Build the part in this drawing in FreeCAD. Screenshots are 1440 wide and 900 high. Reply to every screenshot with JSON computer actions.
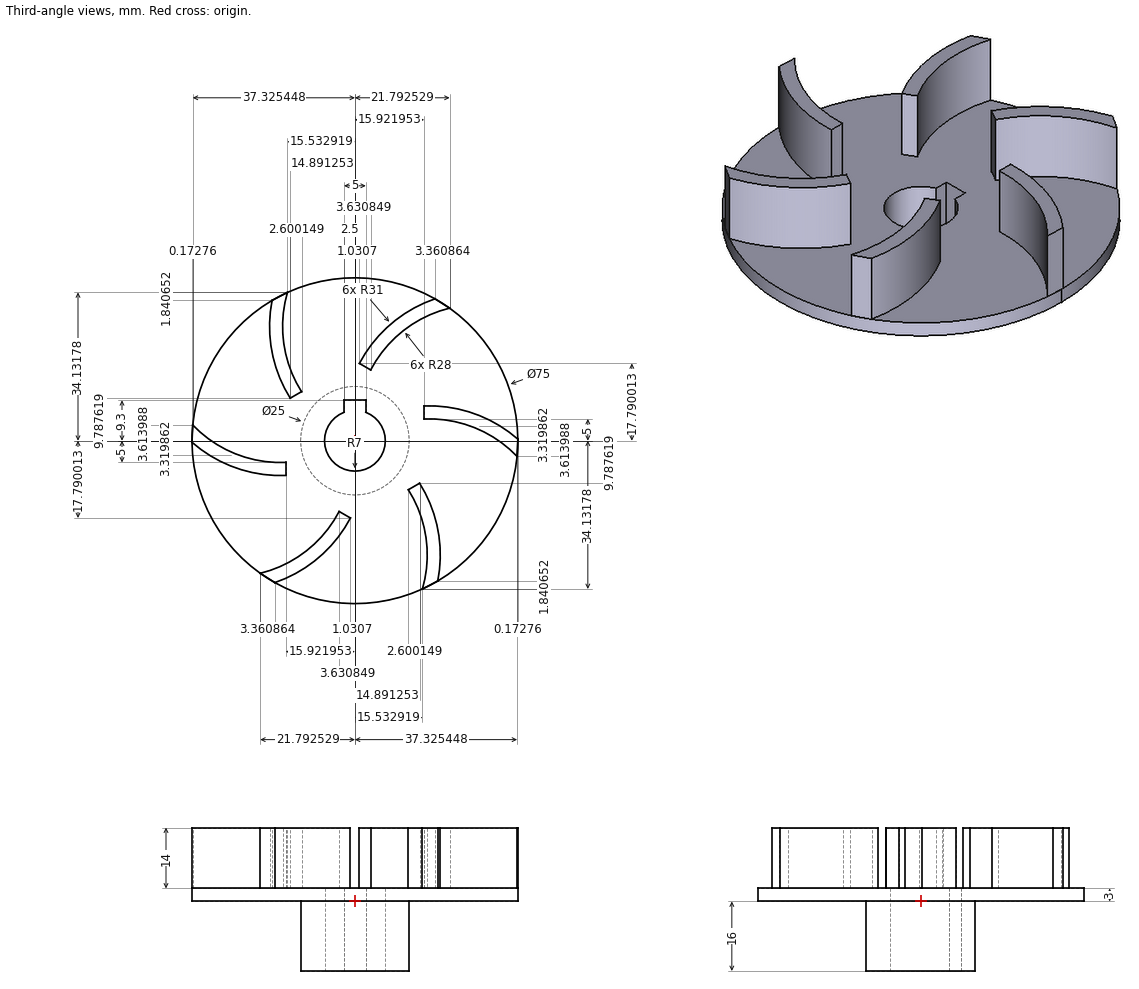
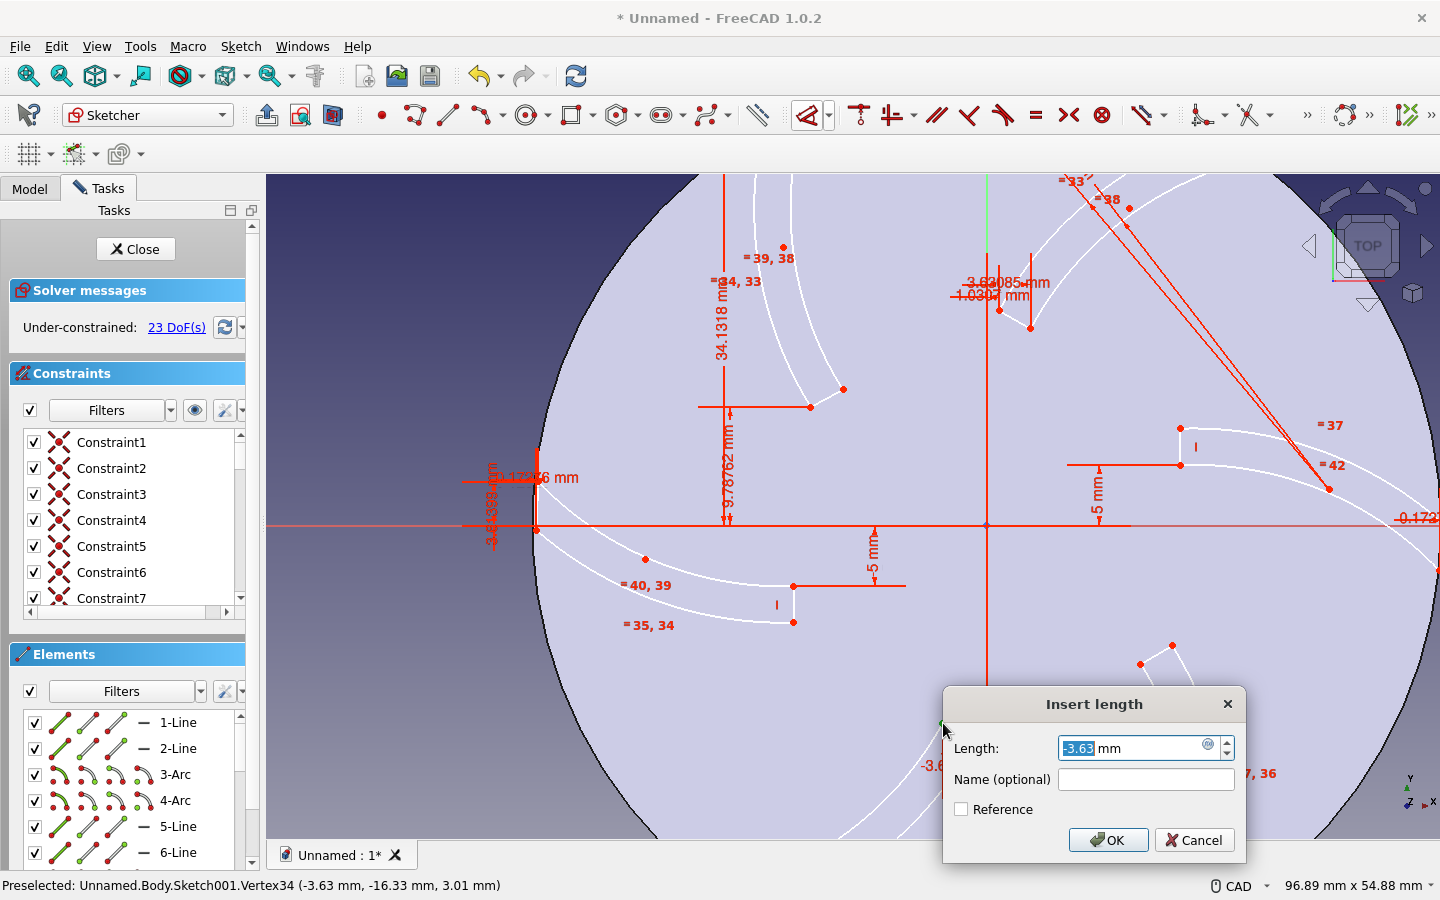
{"action": "type", "text": "-3.630849"}
{"action": "key", "text": "Return"}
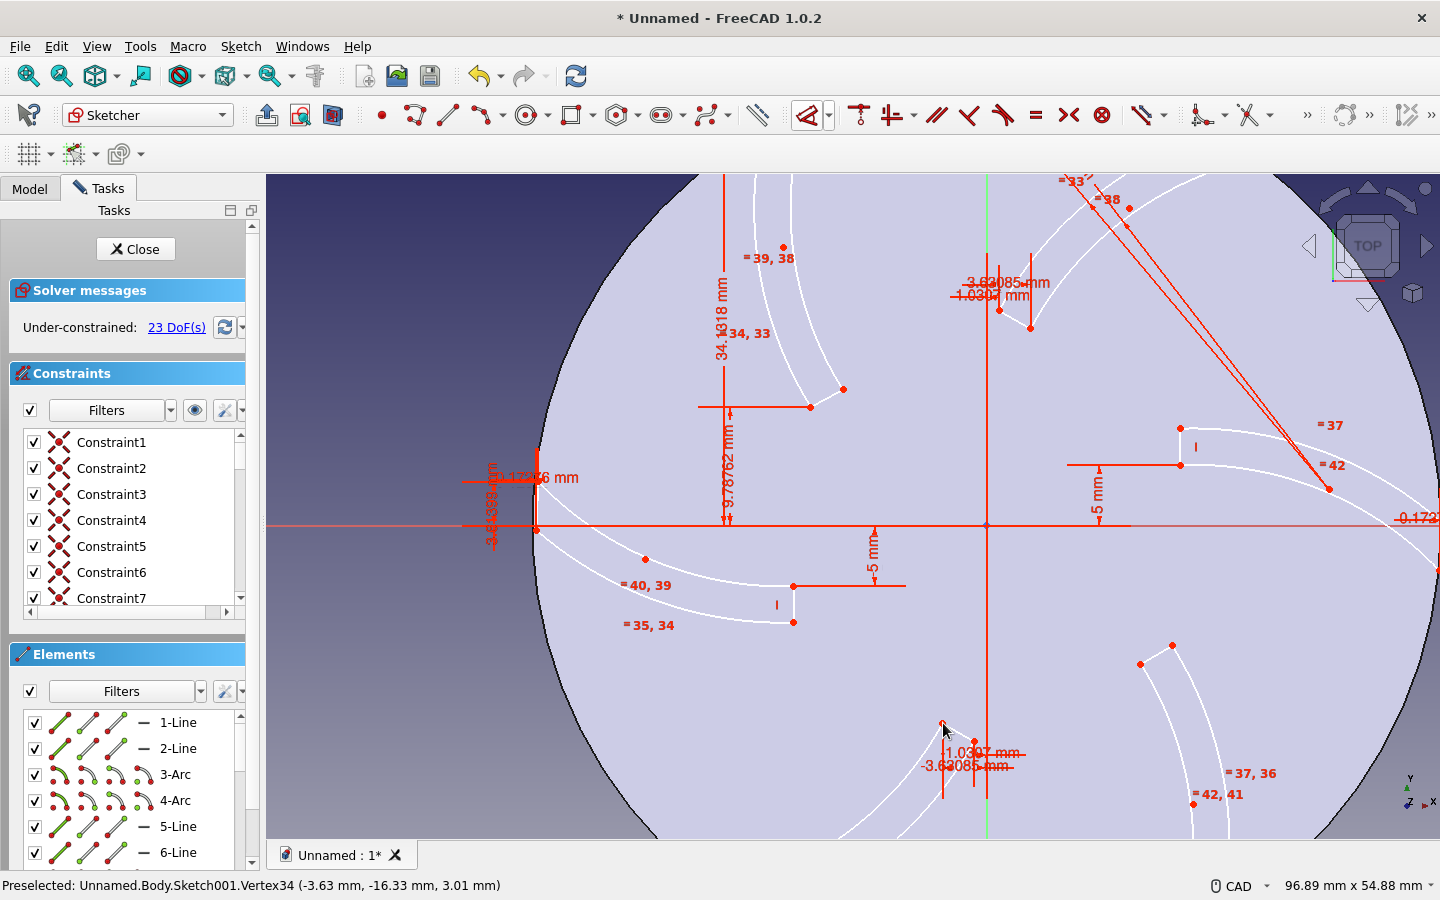
{"action": "scroll", "coordinate": [539, 483], "scroll_direction": "down", "scroll_amount": 3}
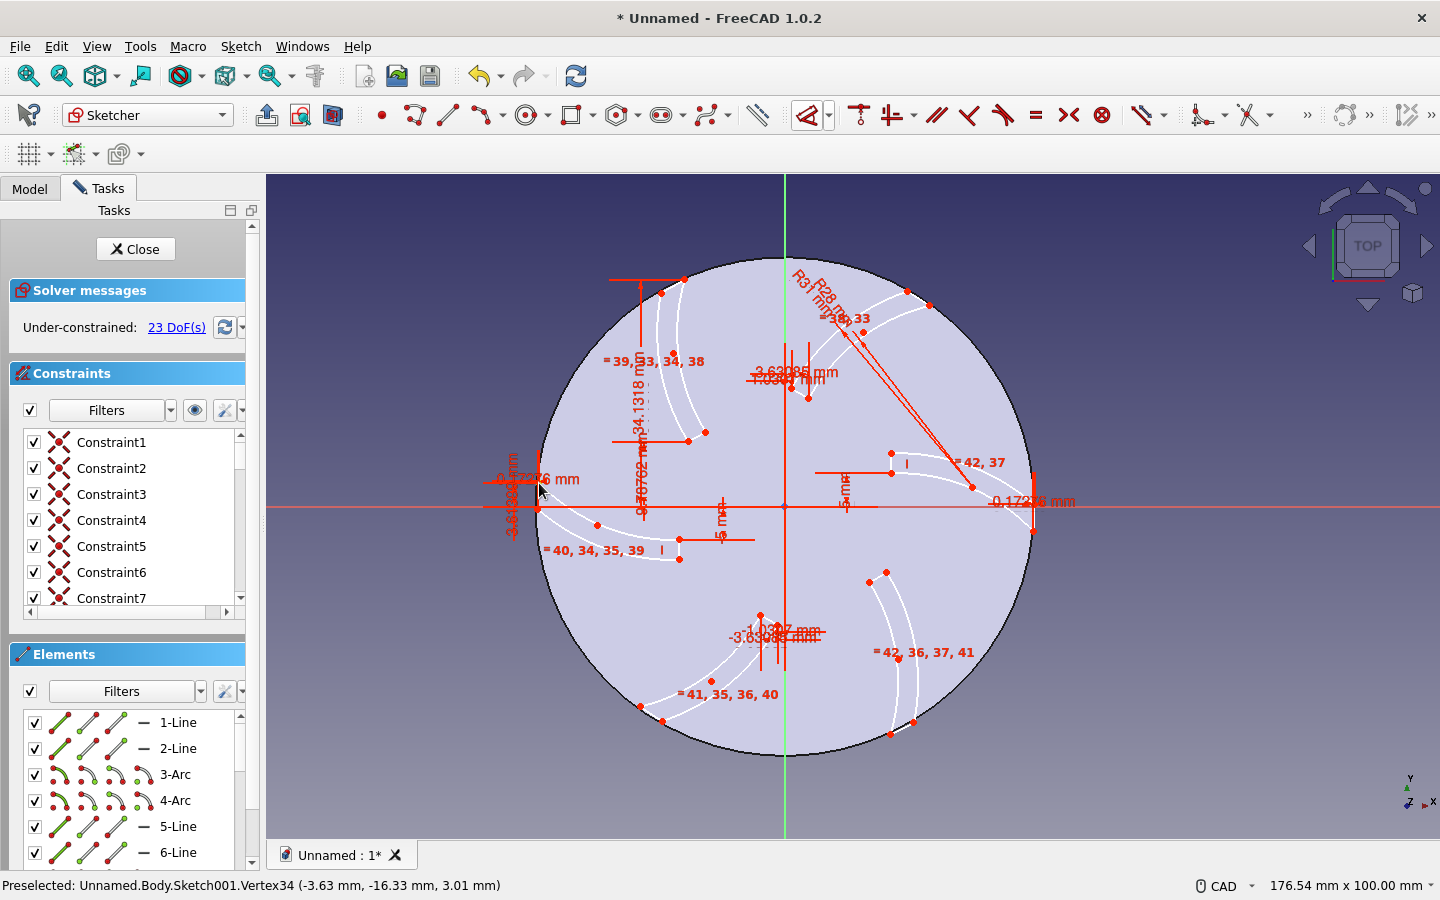
{"action": "left_click", "coordinate": [890, 735]}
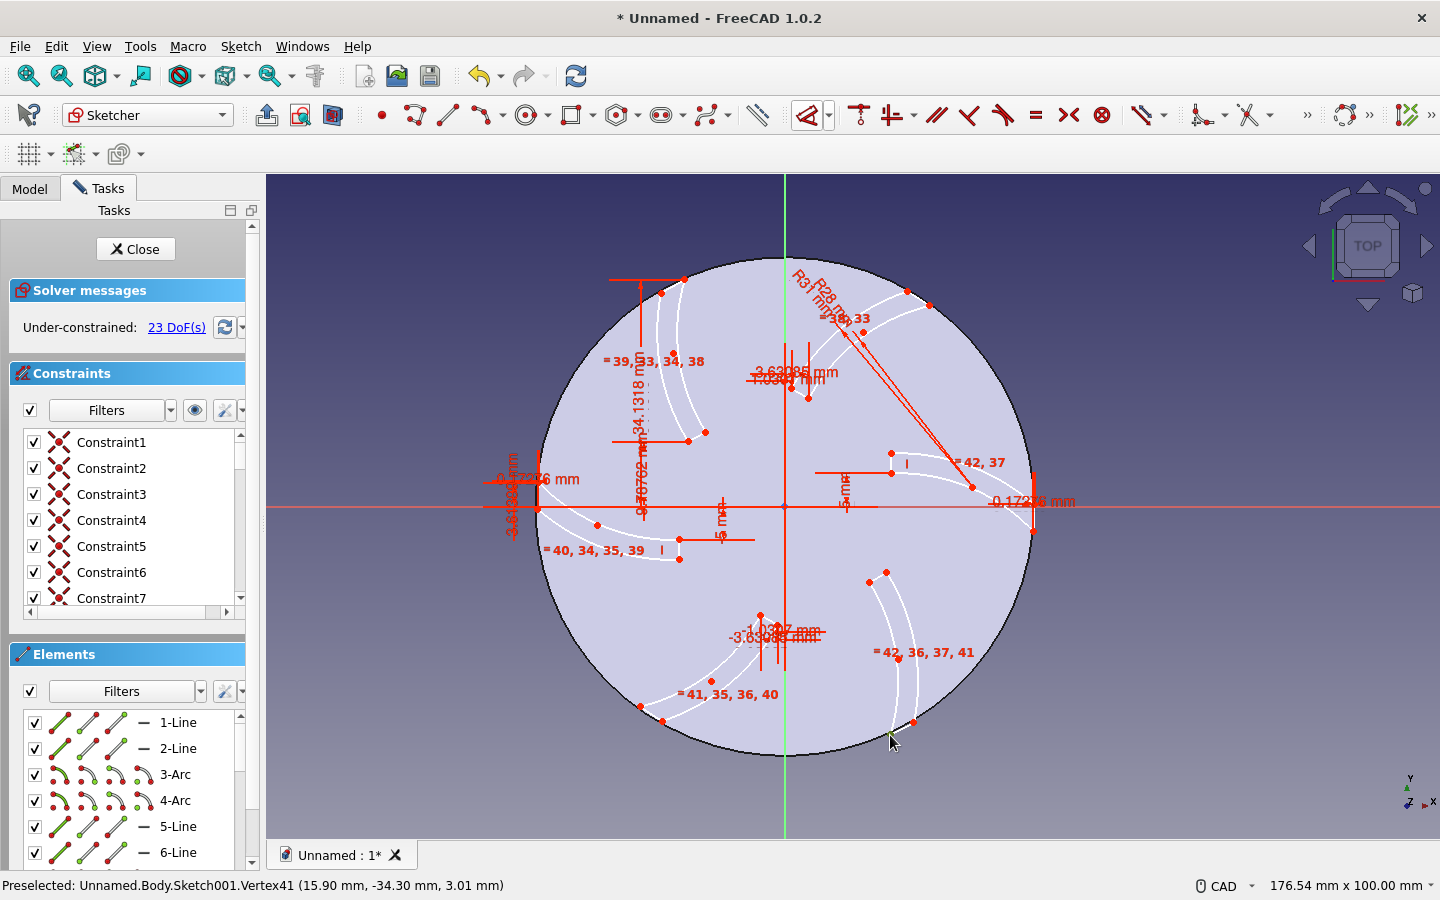
{"action": "key", "text": "i"}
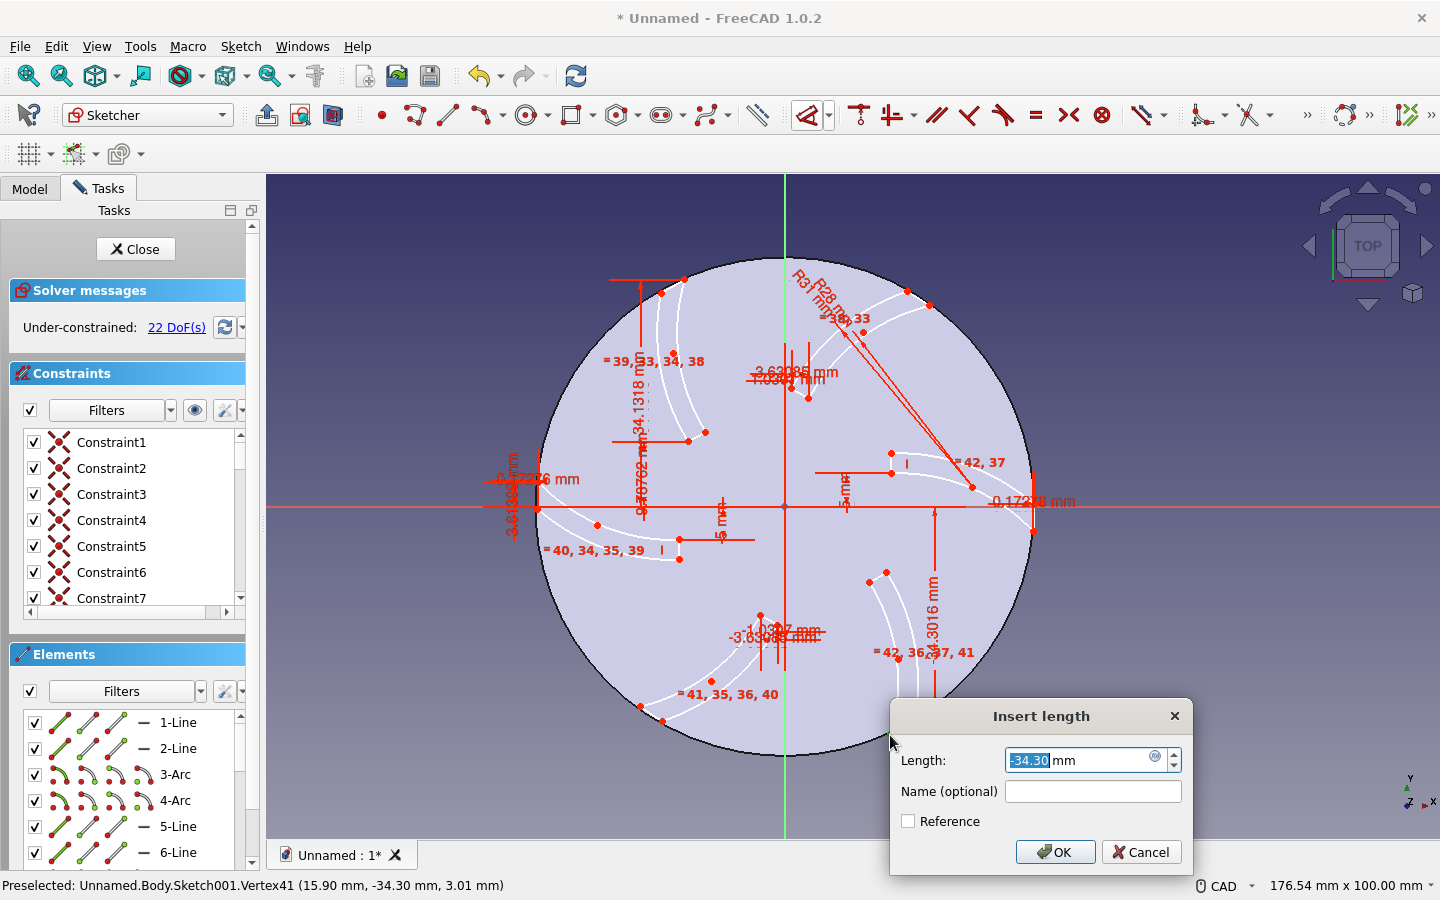
{"action": "type", "text": "-34.13178"}
{"action": "key", "text": "Return"}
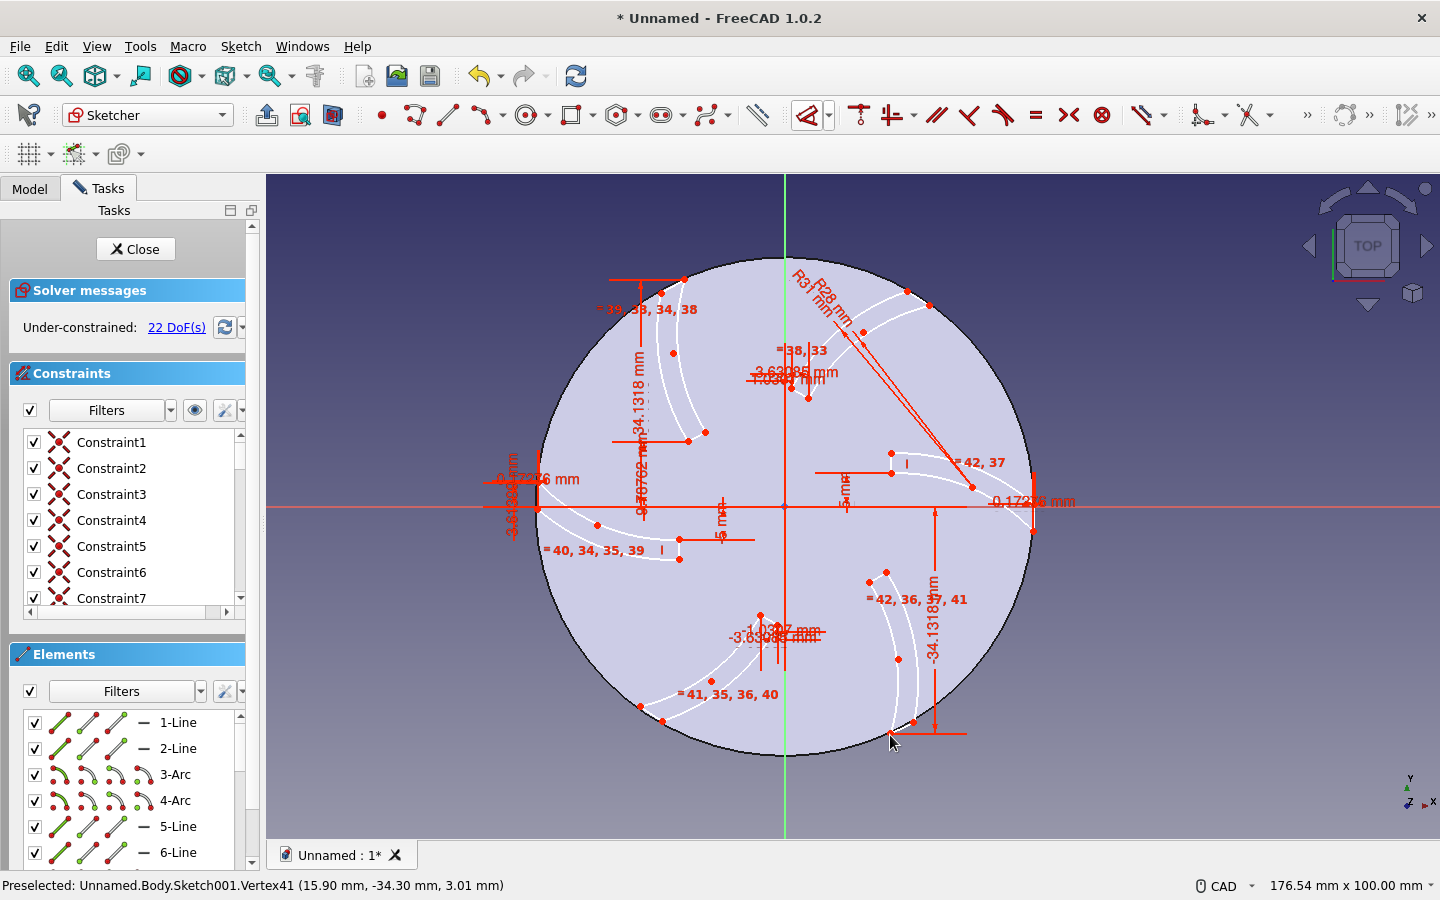
{"action": "left_click", "coordinate": [887, 573]}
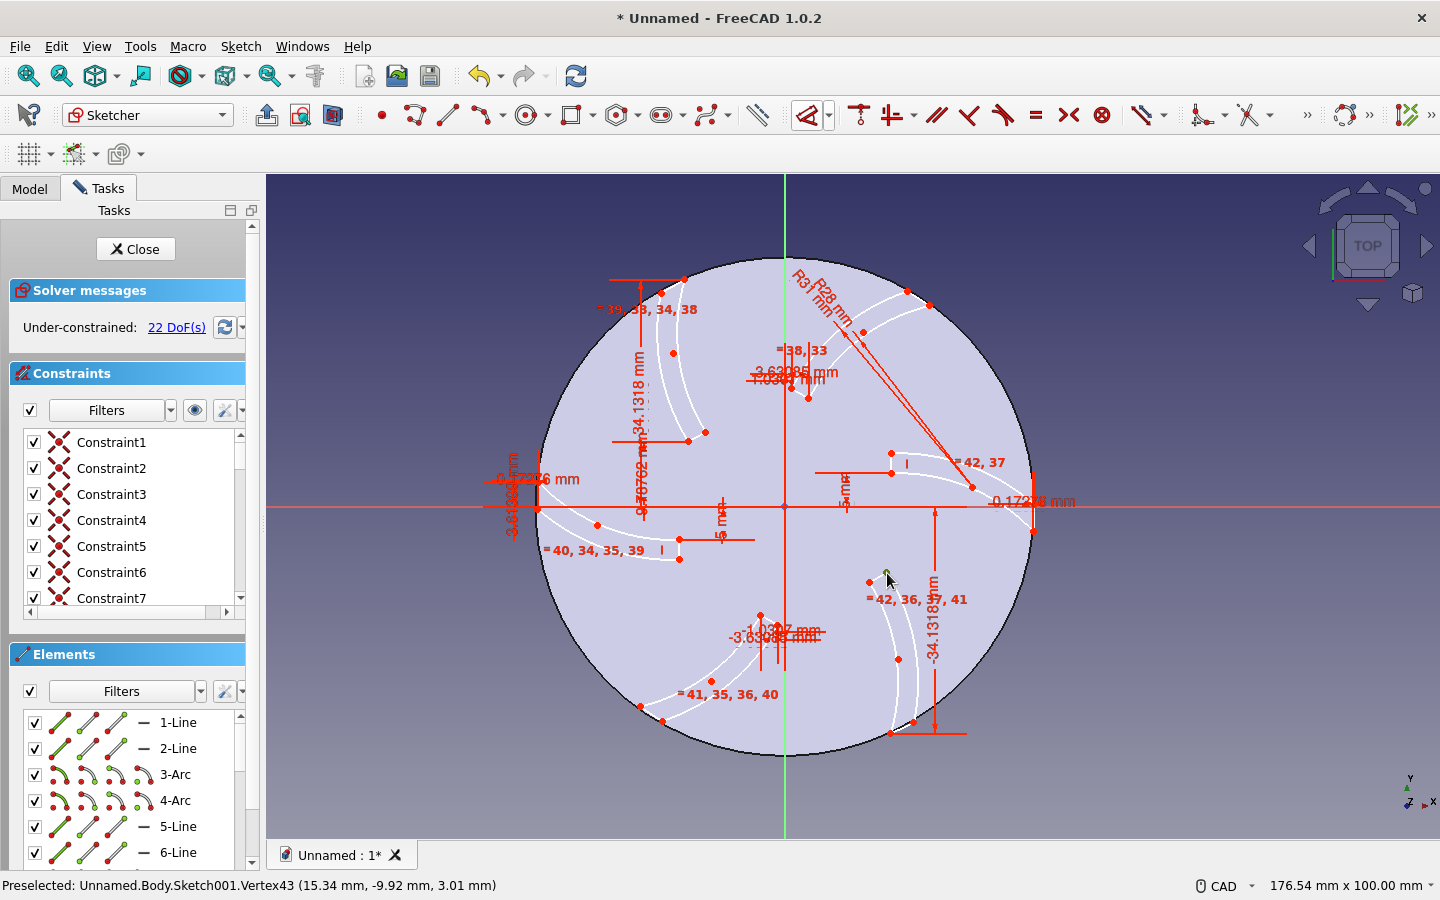
{"action": "key", "text": "i"}